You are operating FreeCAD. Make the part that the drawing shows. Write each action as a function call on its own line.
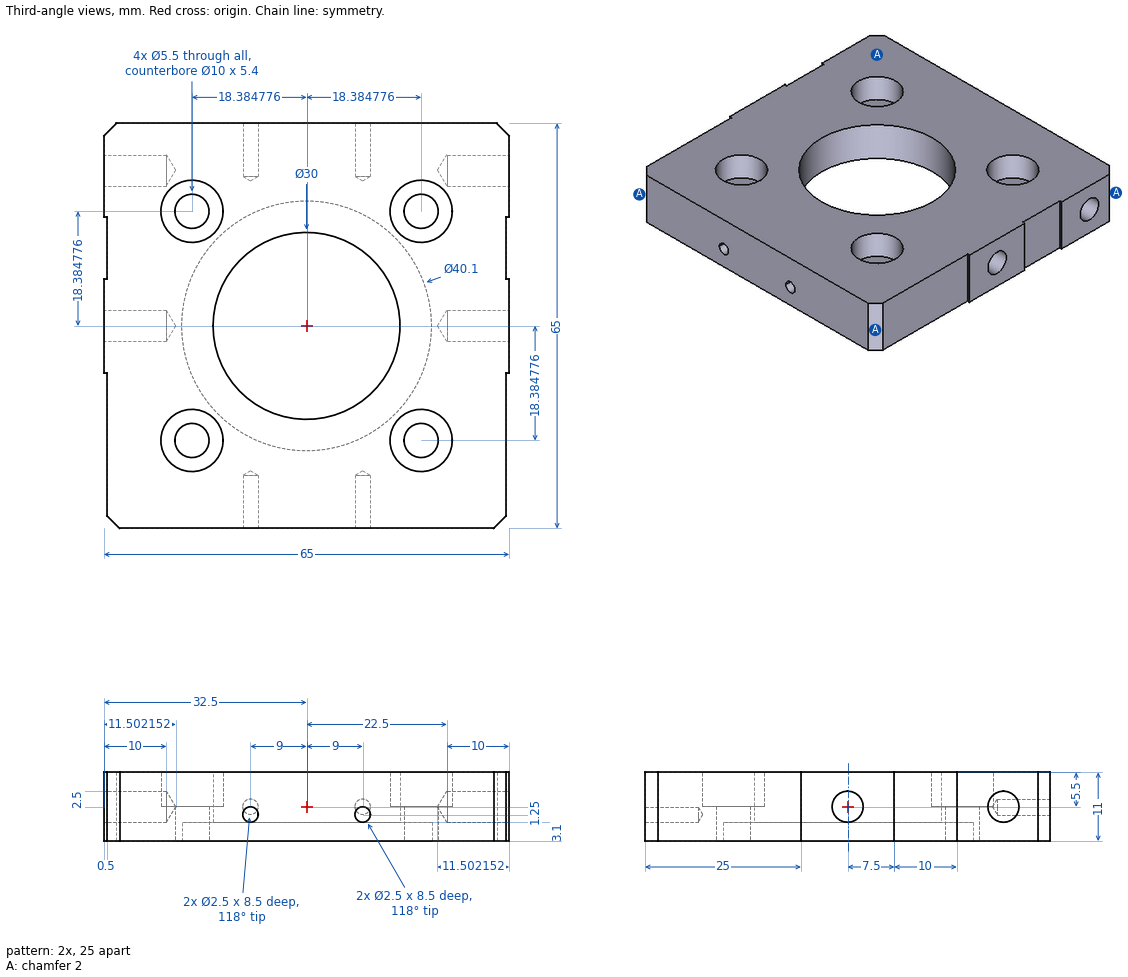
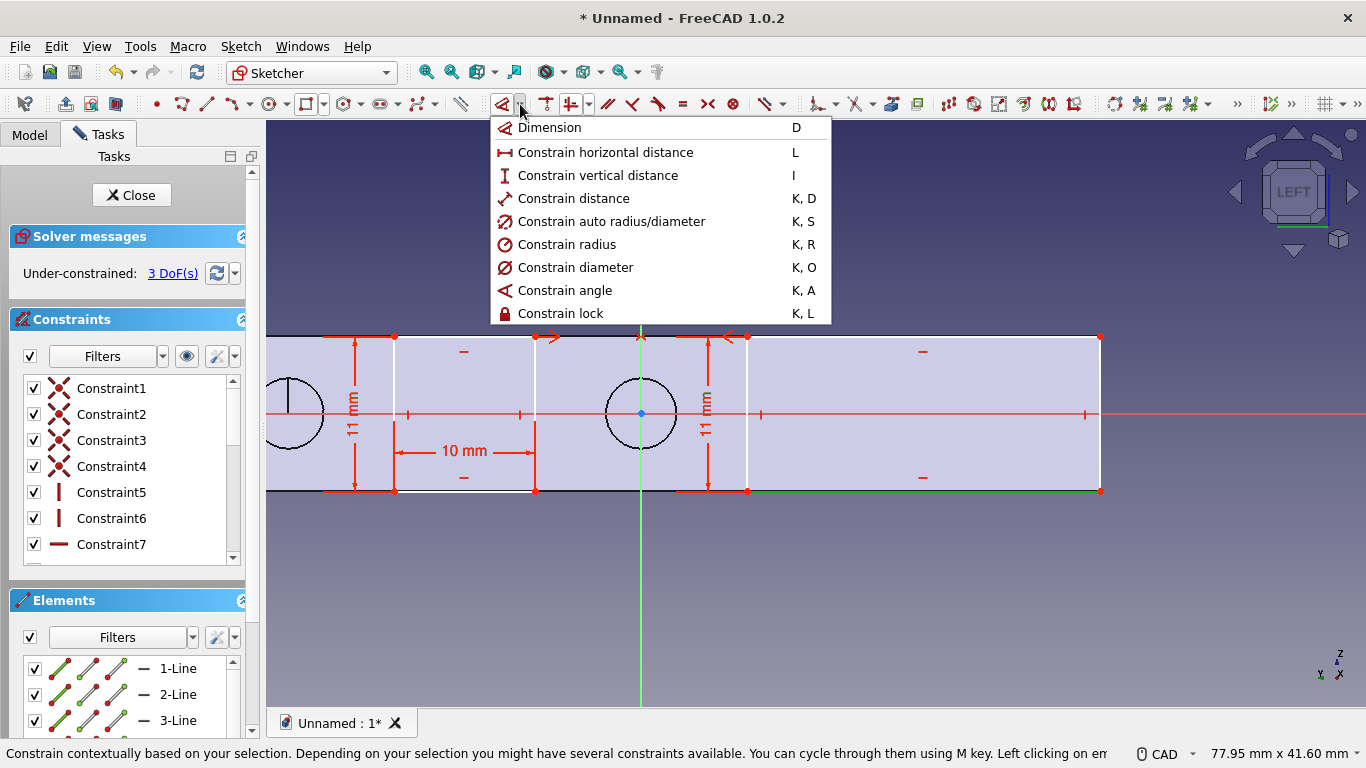
click(661, 152)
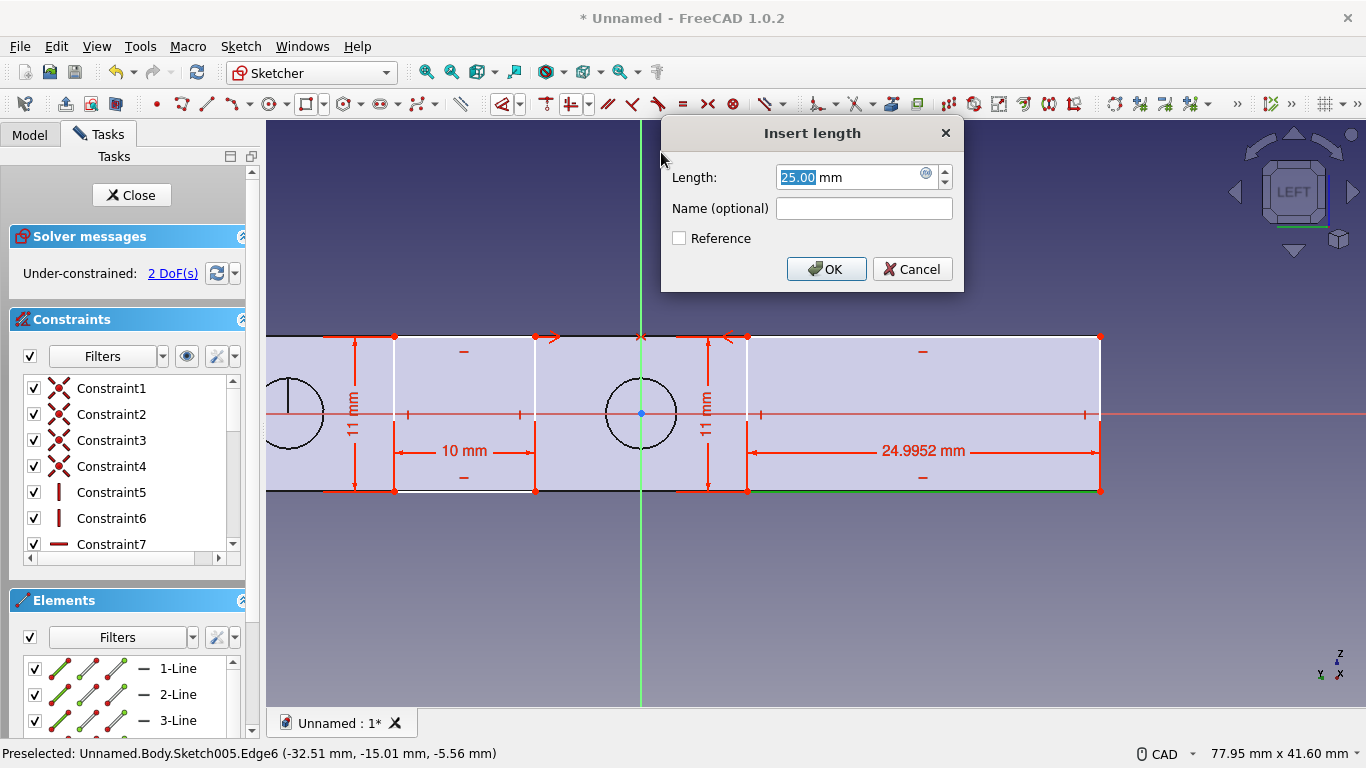
text(25)
key(Return)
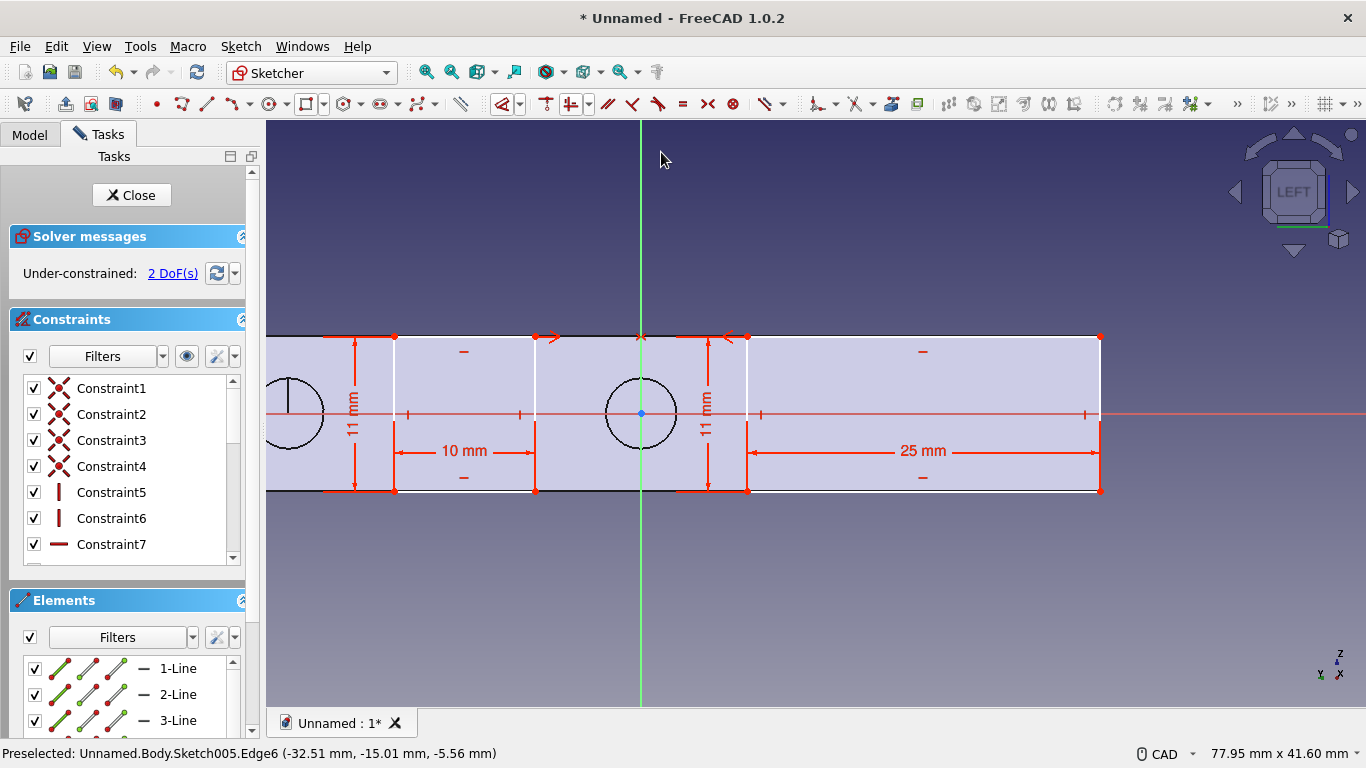
click(394, 337)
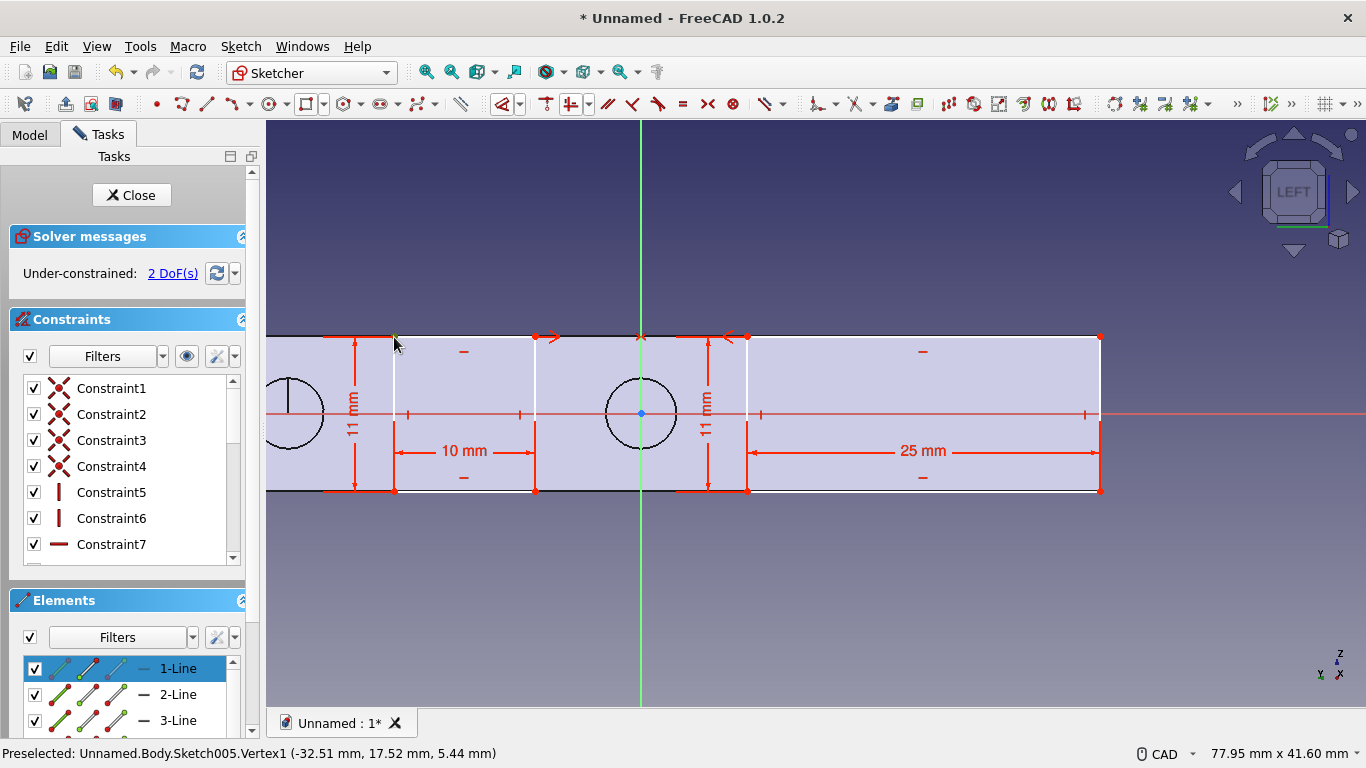
click(520, 104)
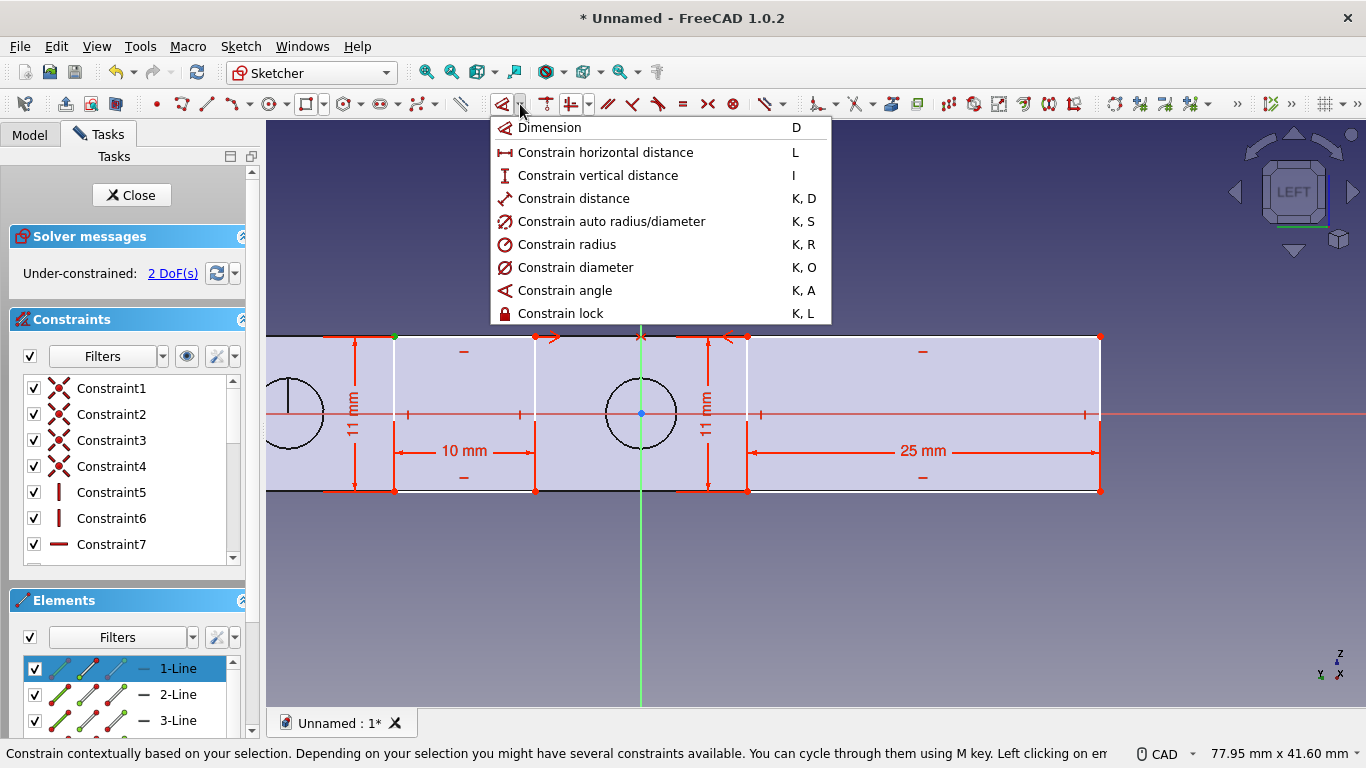
click(661, 176)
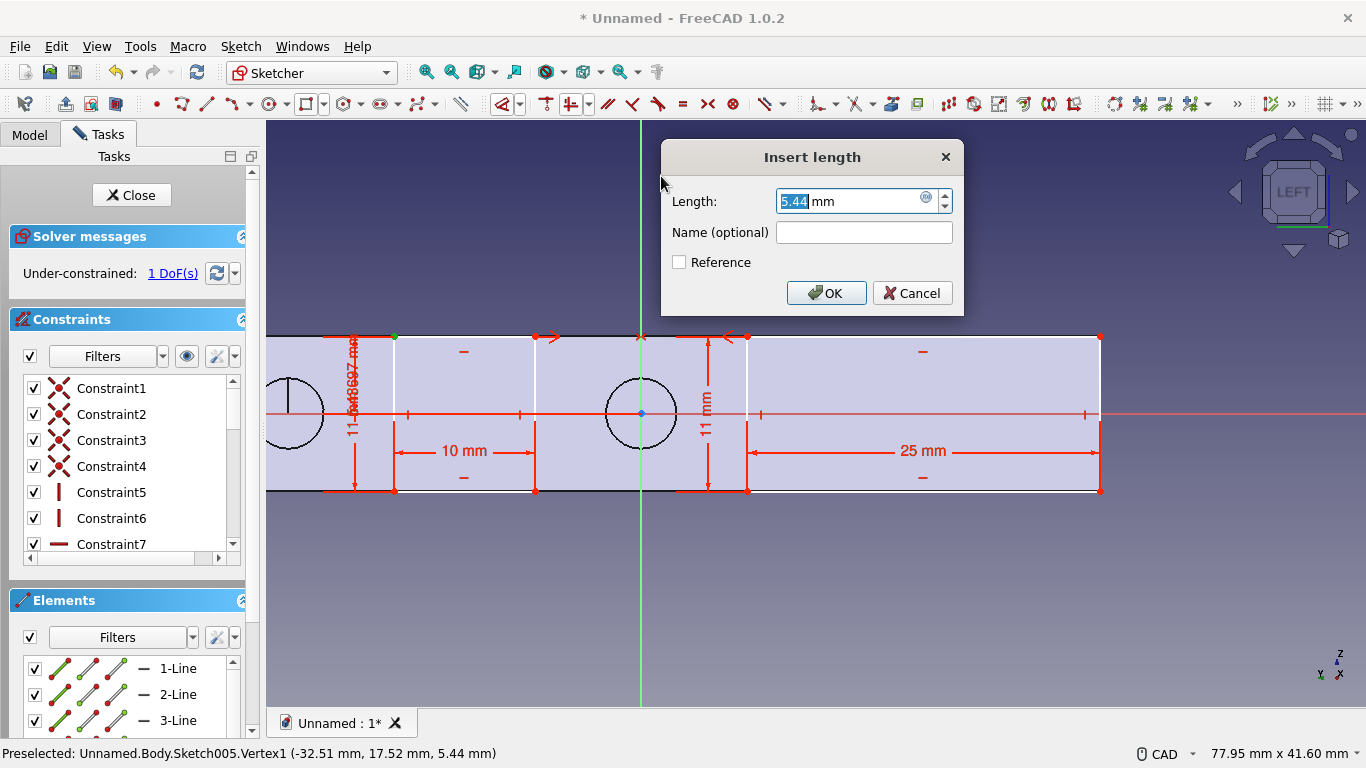
text(5.5)
key(Return)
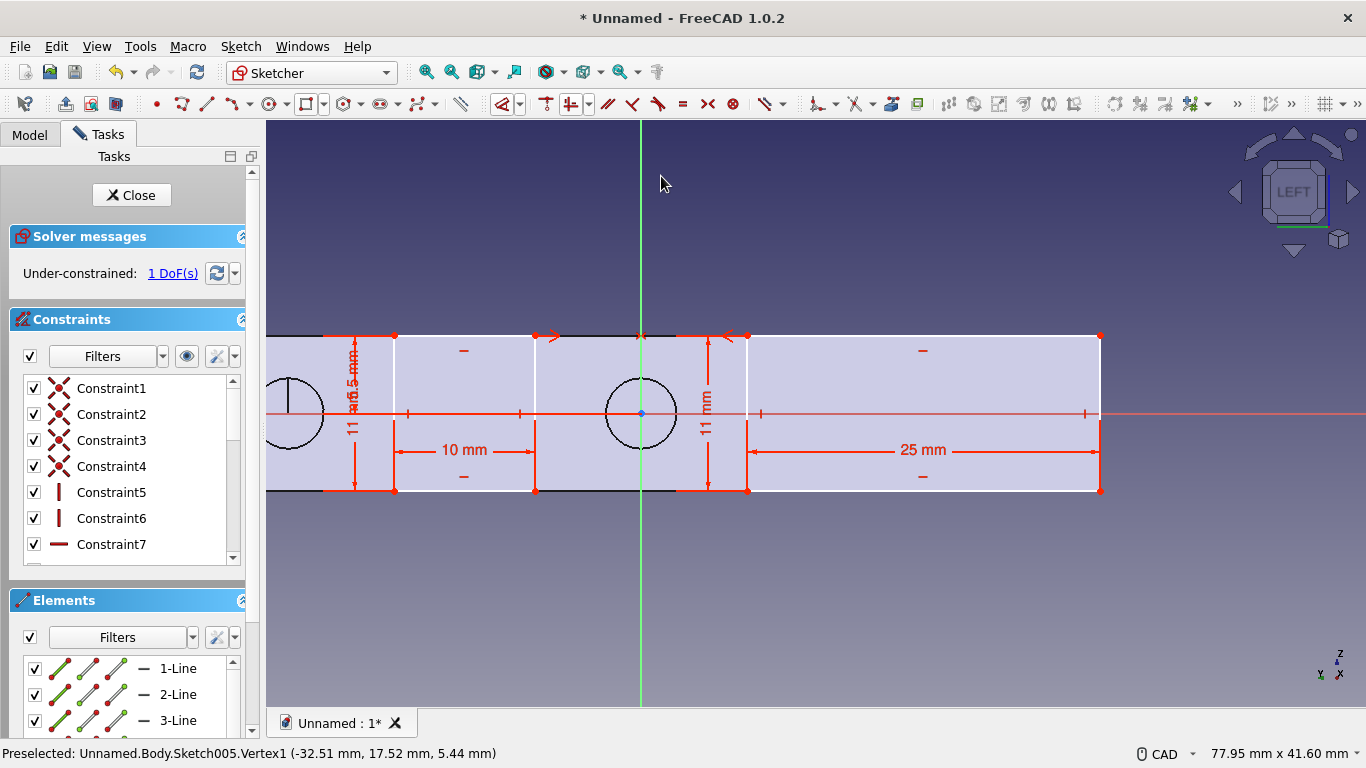
click(535, 491)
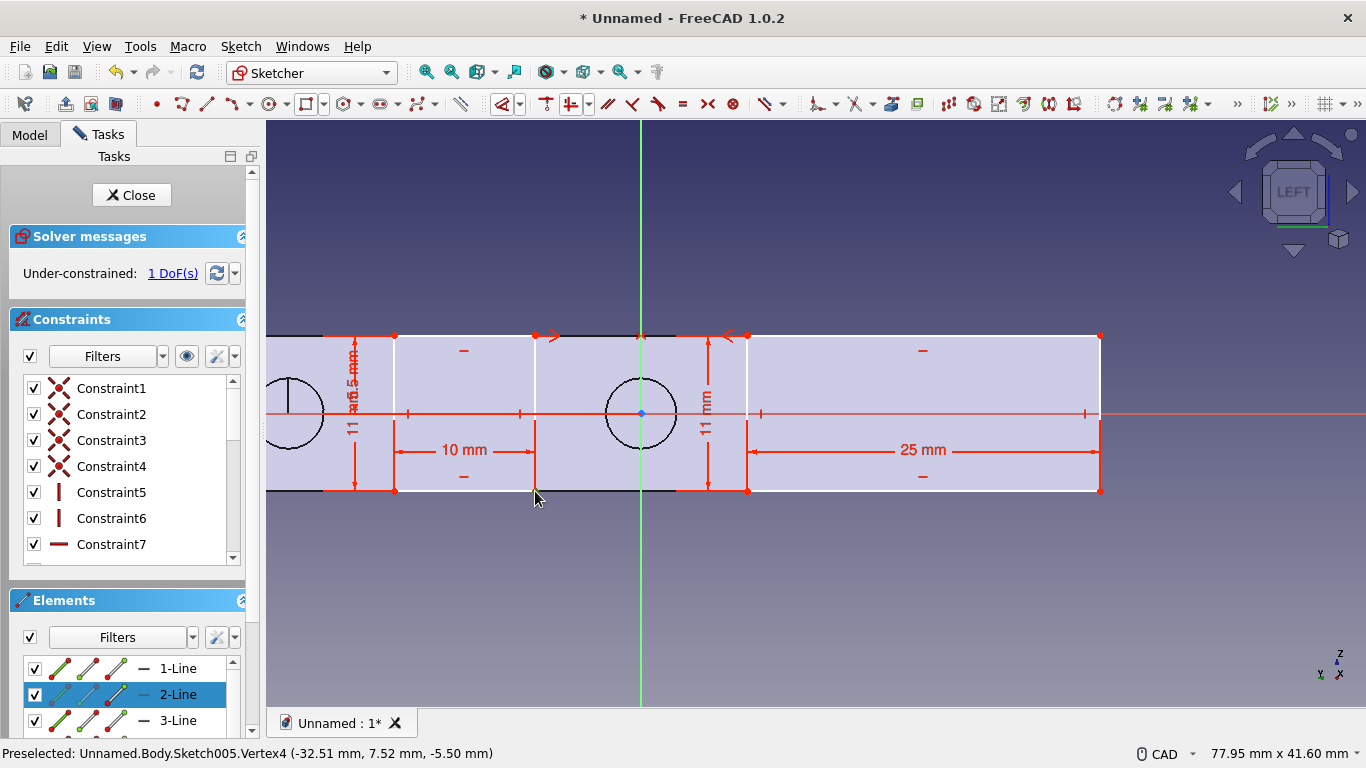
click(520, 104)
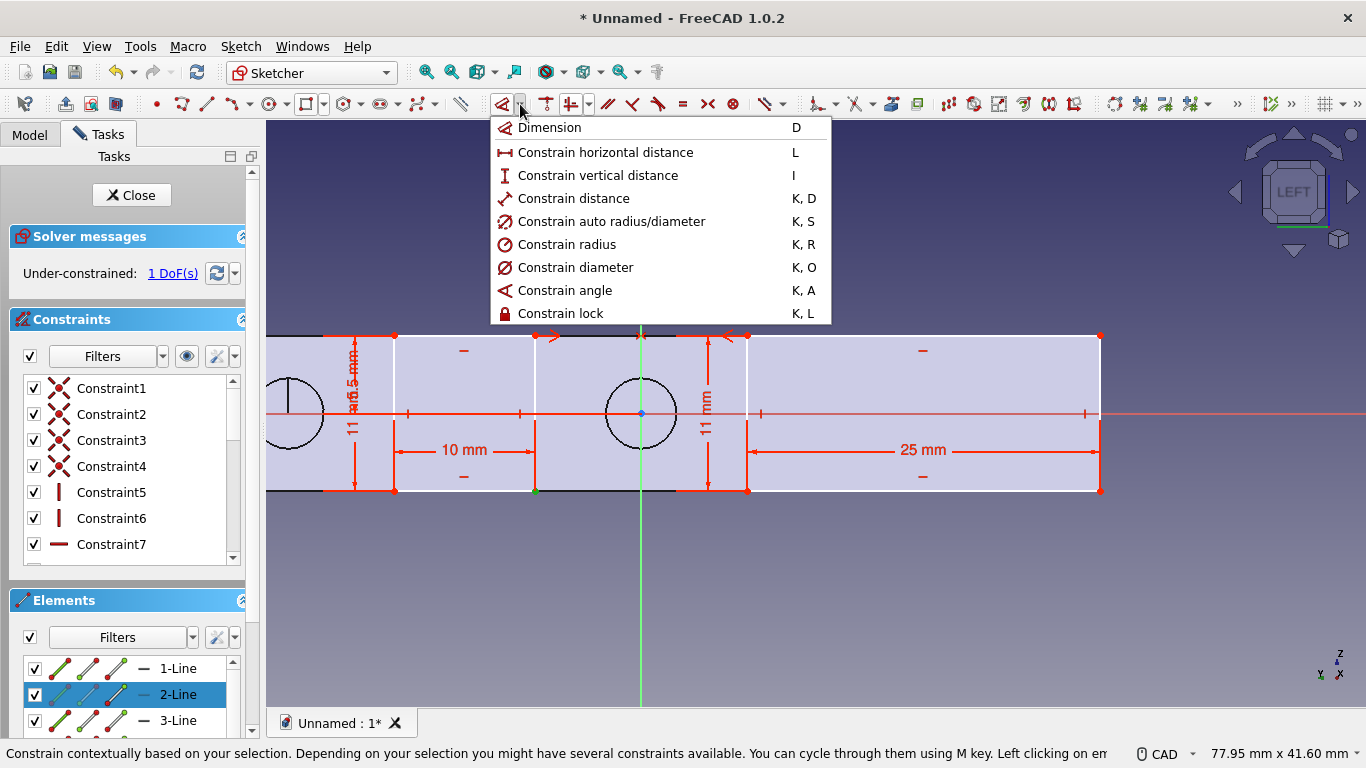
click(661, 152)